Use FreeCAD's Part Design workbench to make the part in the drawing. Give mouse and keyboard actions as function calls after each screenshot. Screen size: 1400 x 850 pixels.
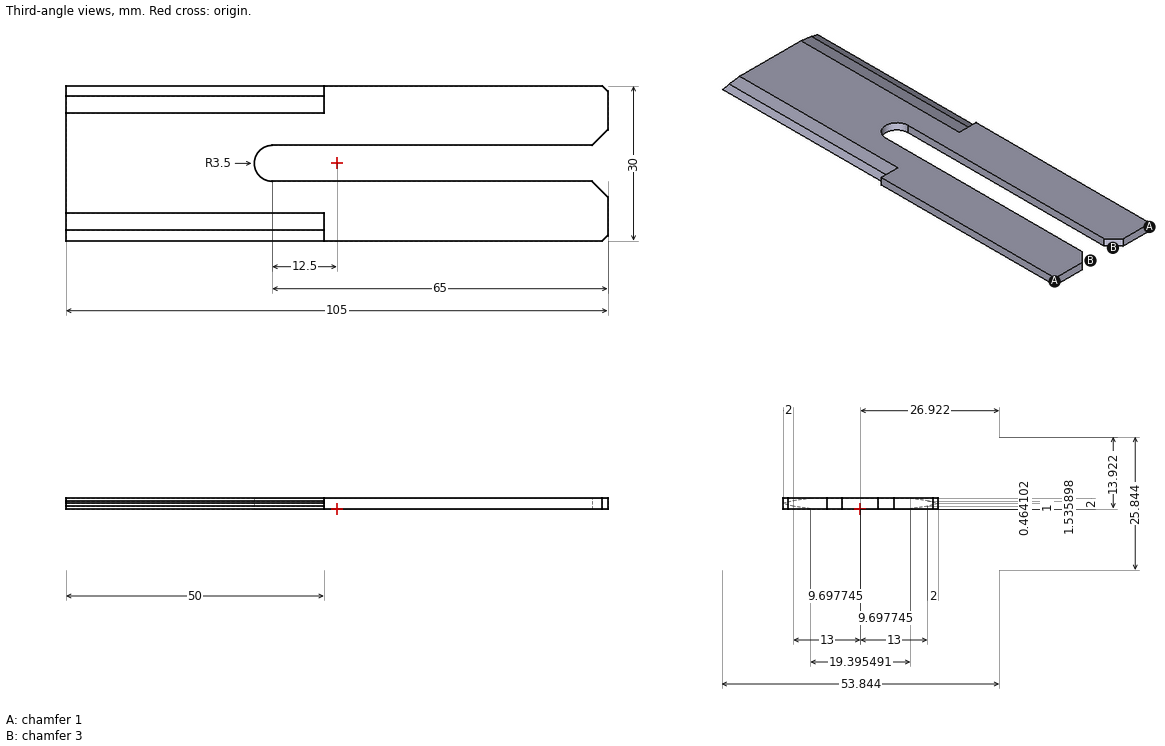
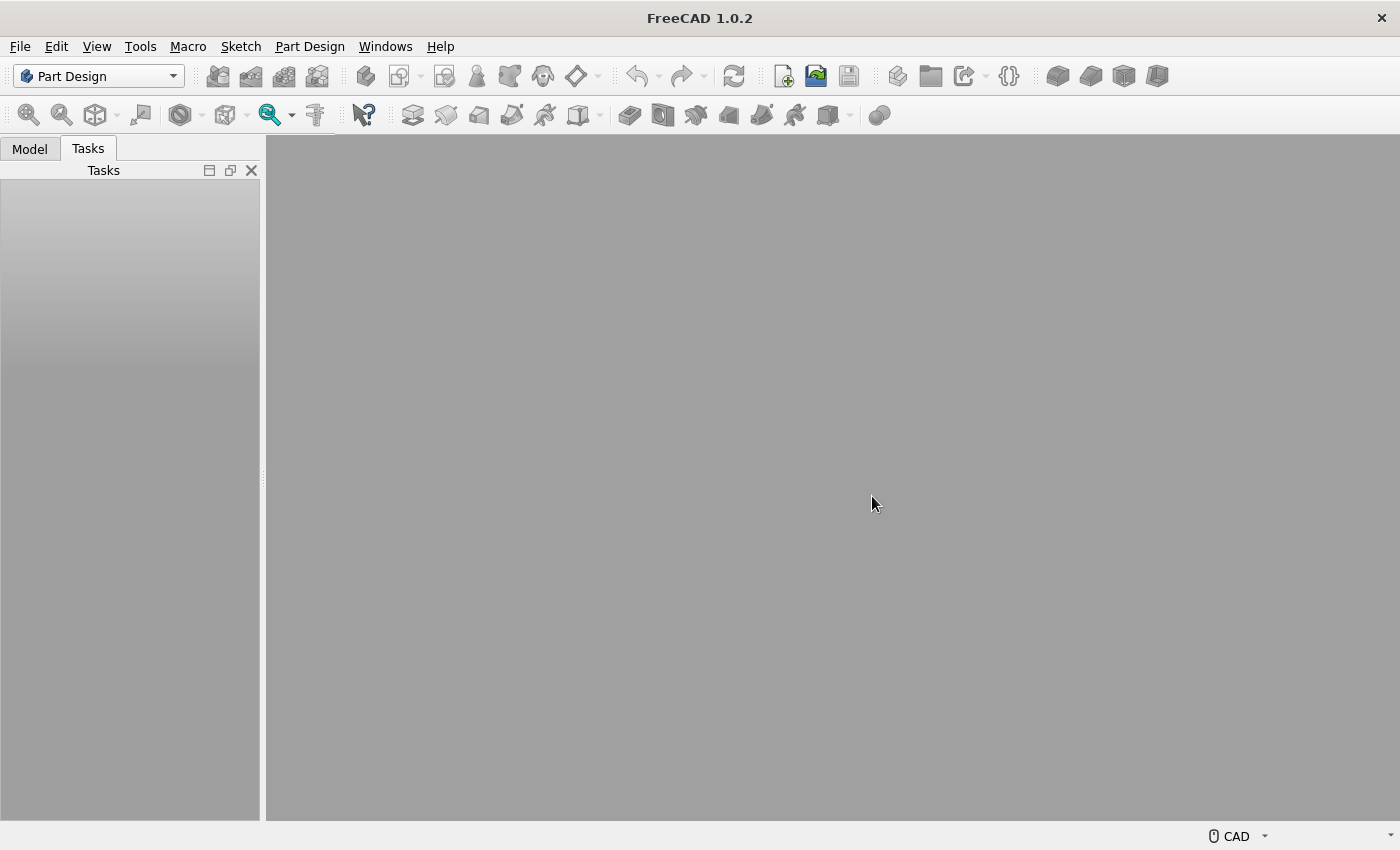
click(783, 76)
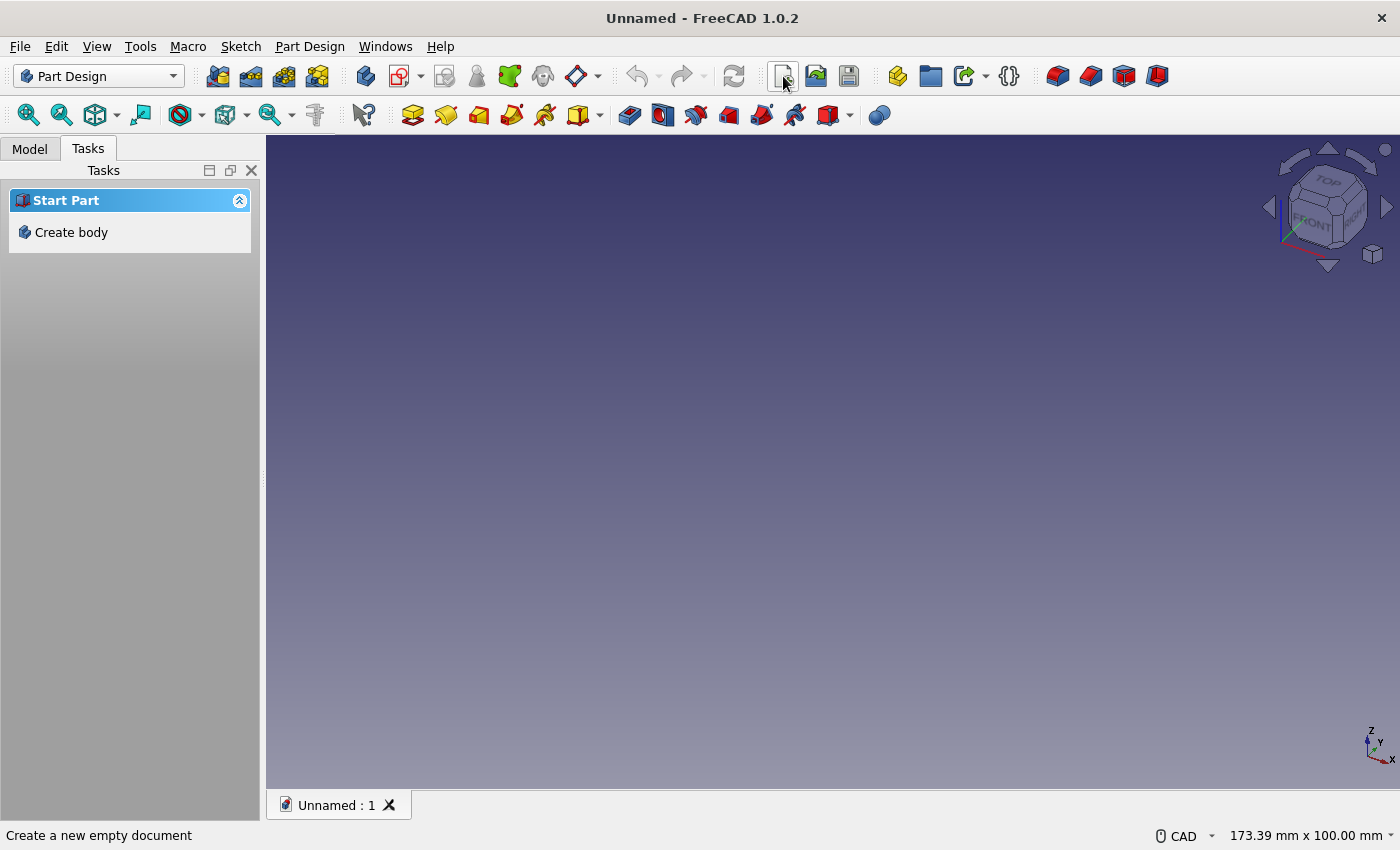
click(398, 76)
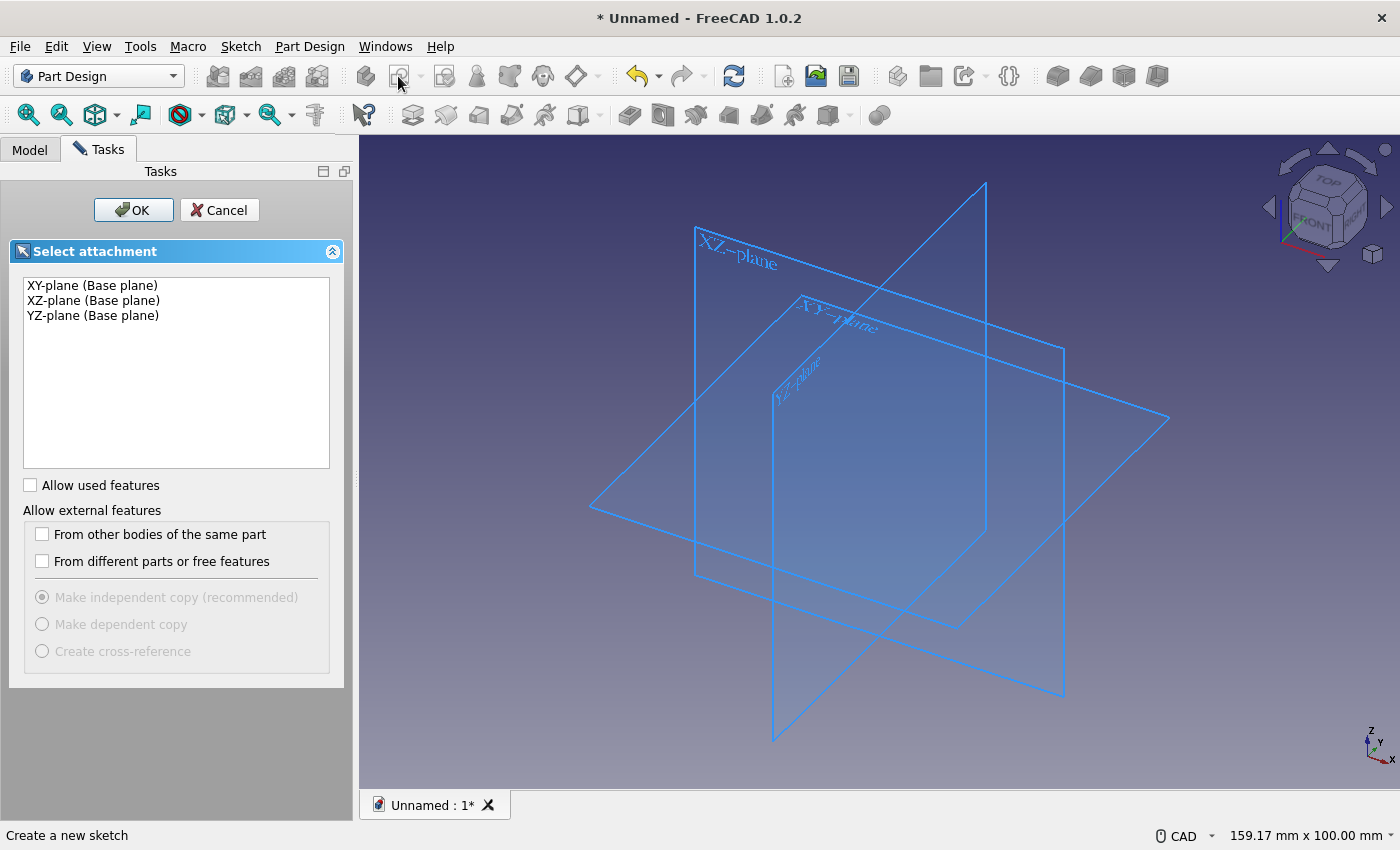
click(84, 286)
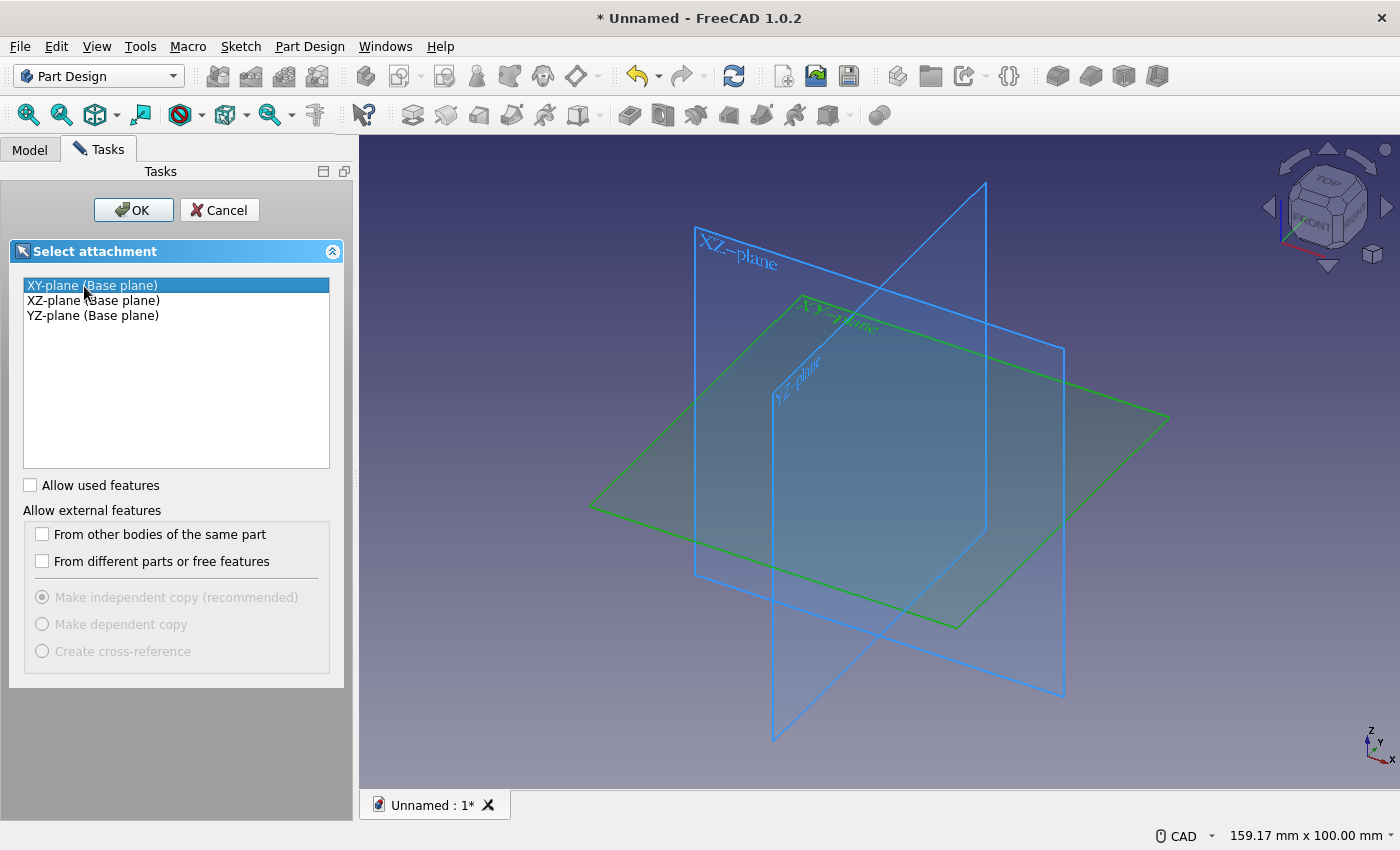
click(134, 210)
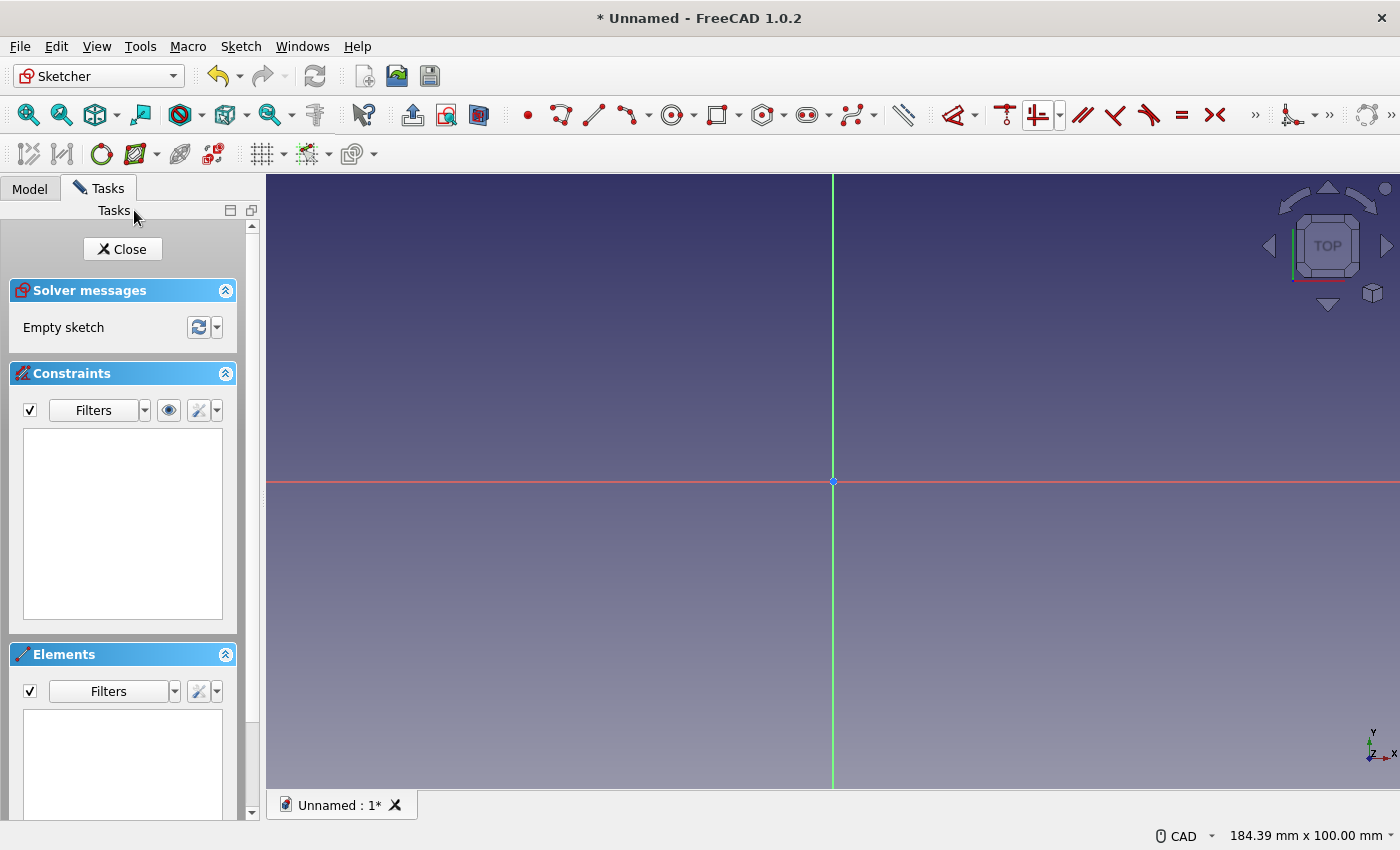
key(g)
key(v)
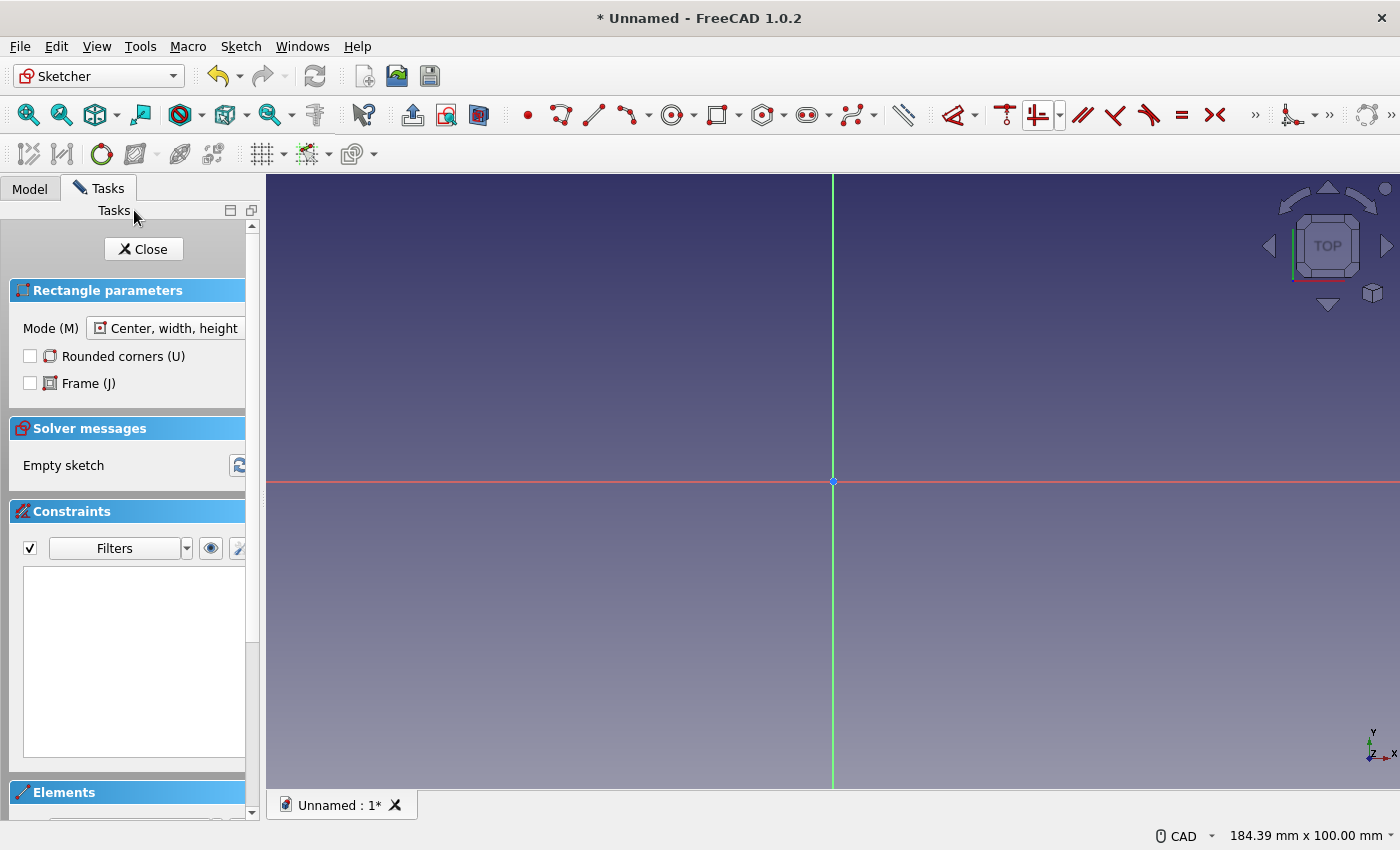
click(833, 482)
click(1156, 389)
key(Escape)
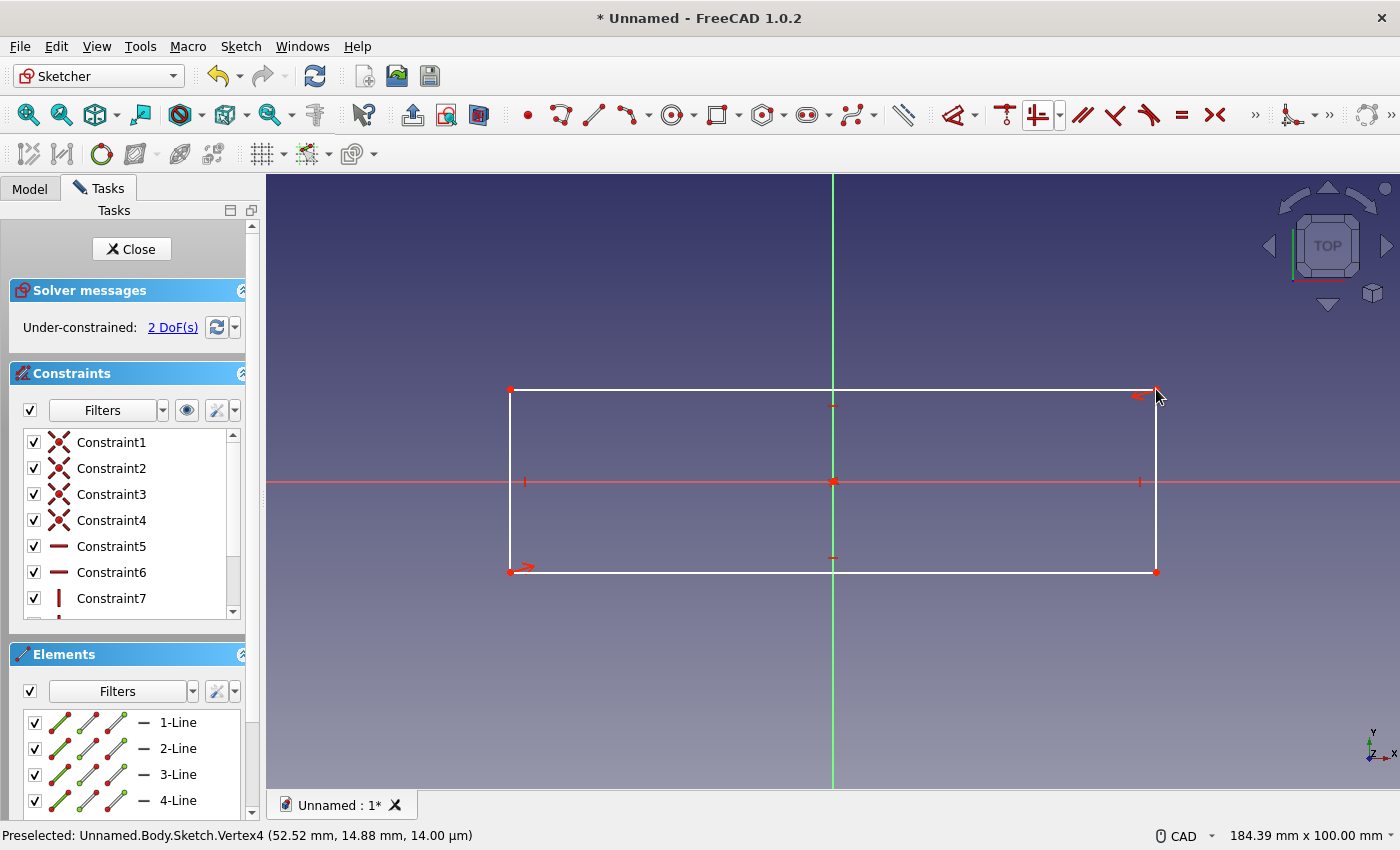
click(952, 116)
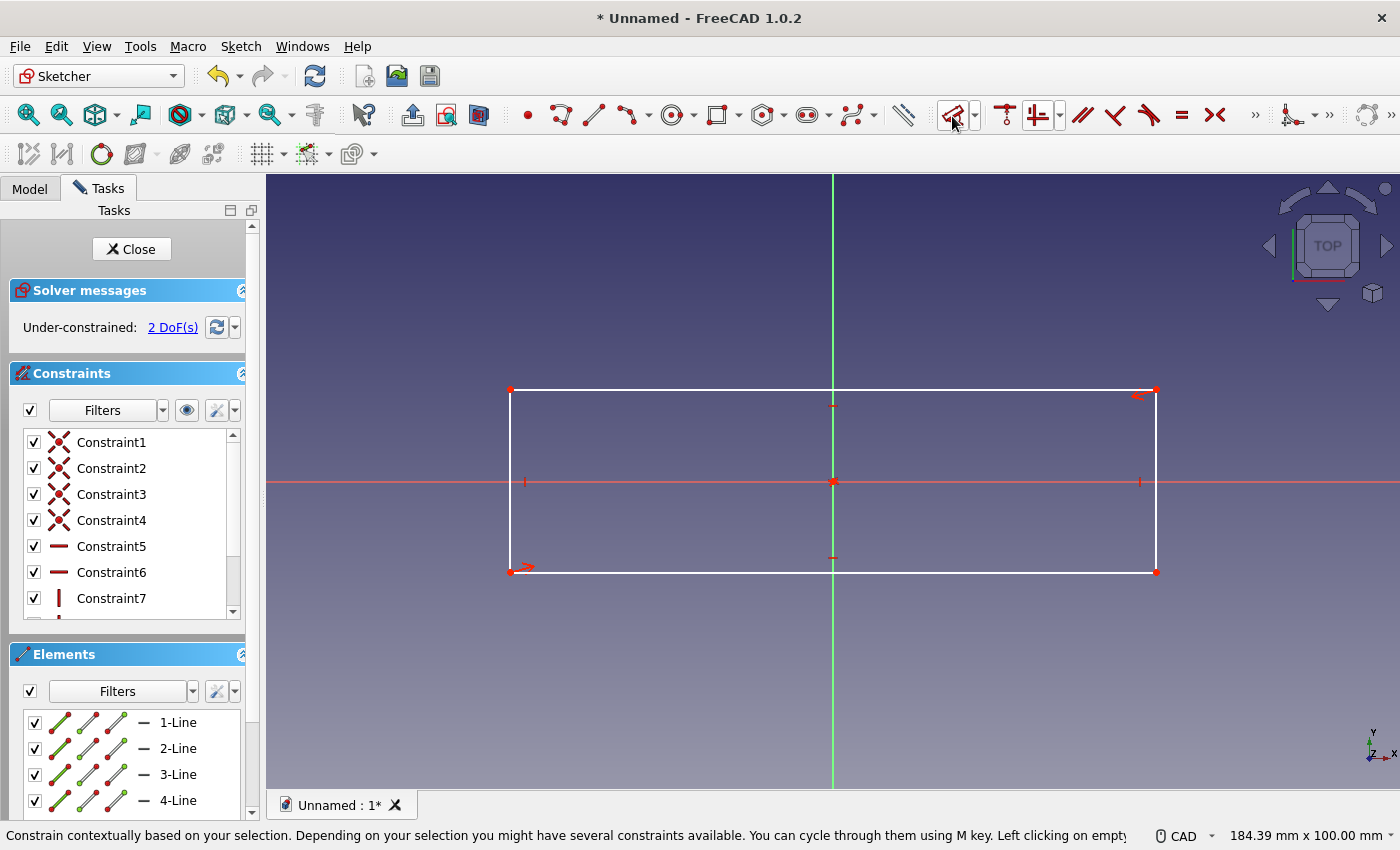
click(1156, 518)
click(1190, 439)